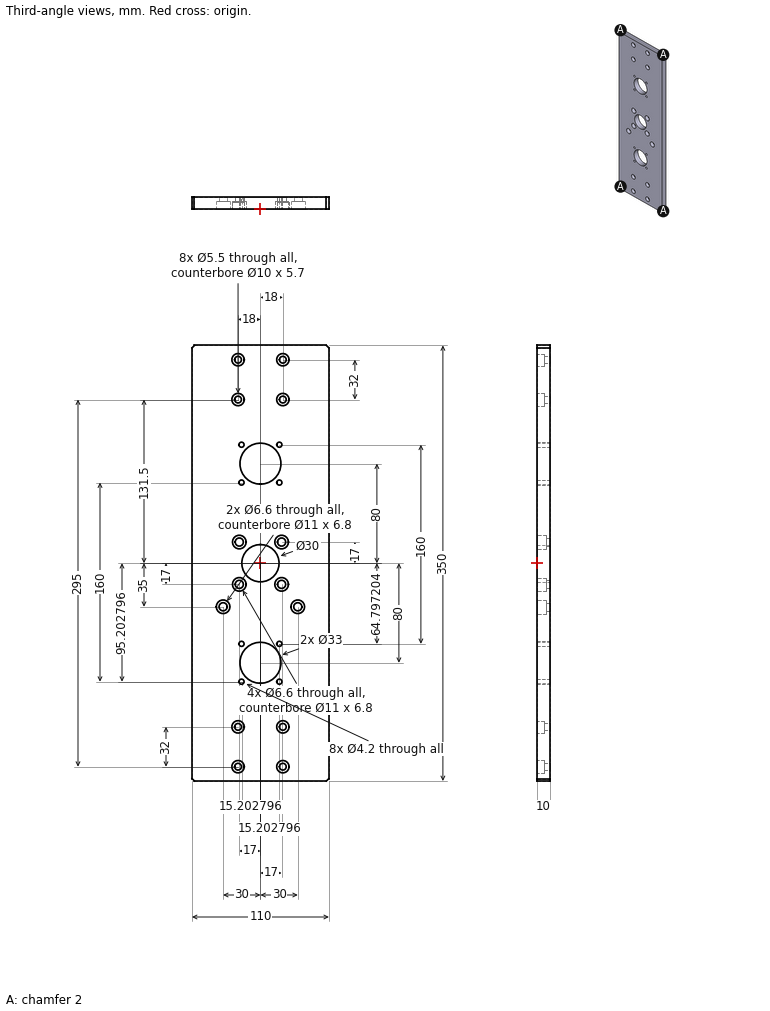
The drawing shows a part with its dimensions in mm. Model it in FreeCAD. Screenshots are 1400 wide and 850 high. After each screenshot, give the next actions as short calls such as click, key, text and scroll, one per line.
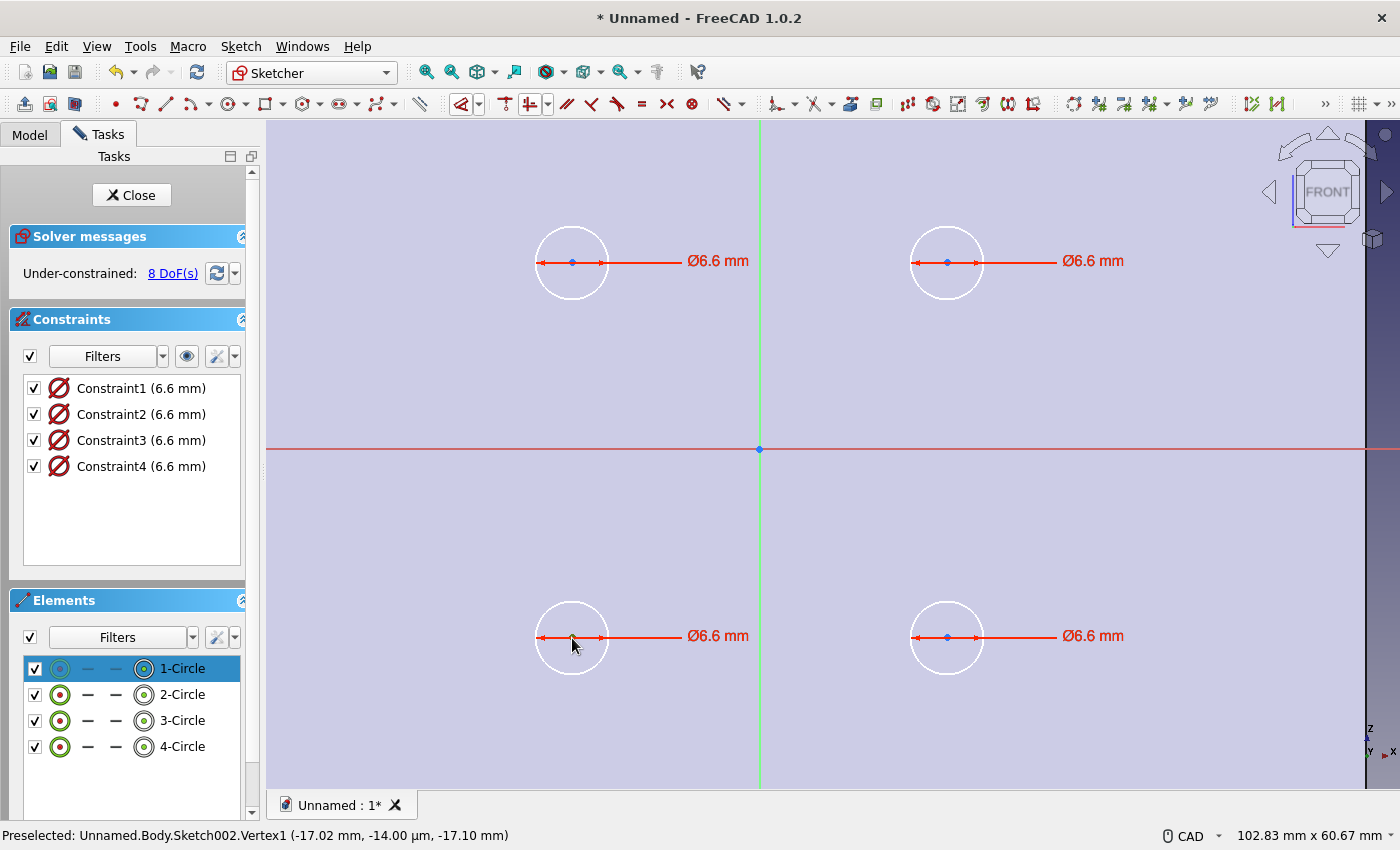
click(947, 638)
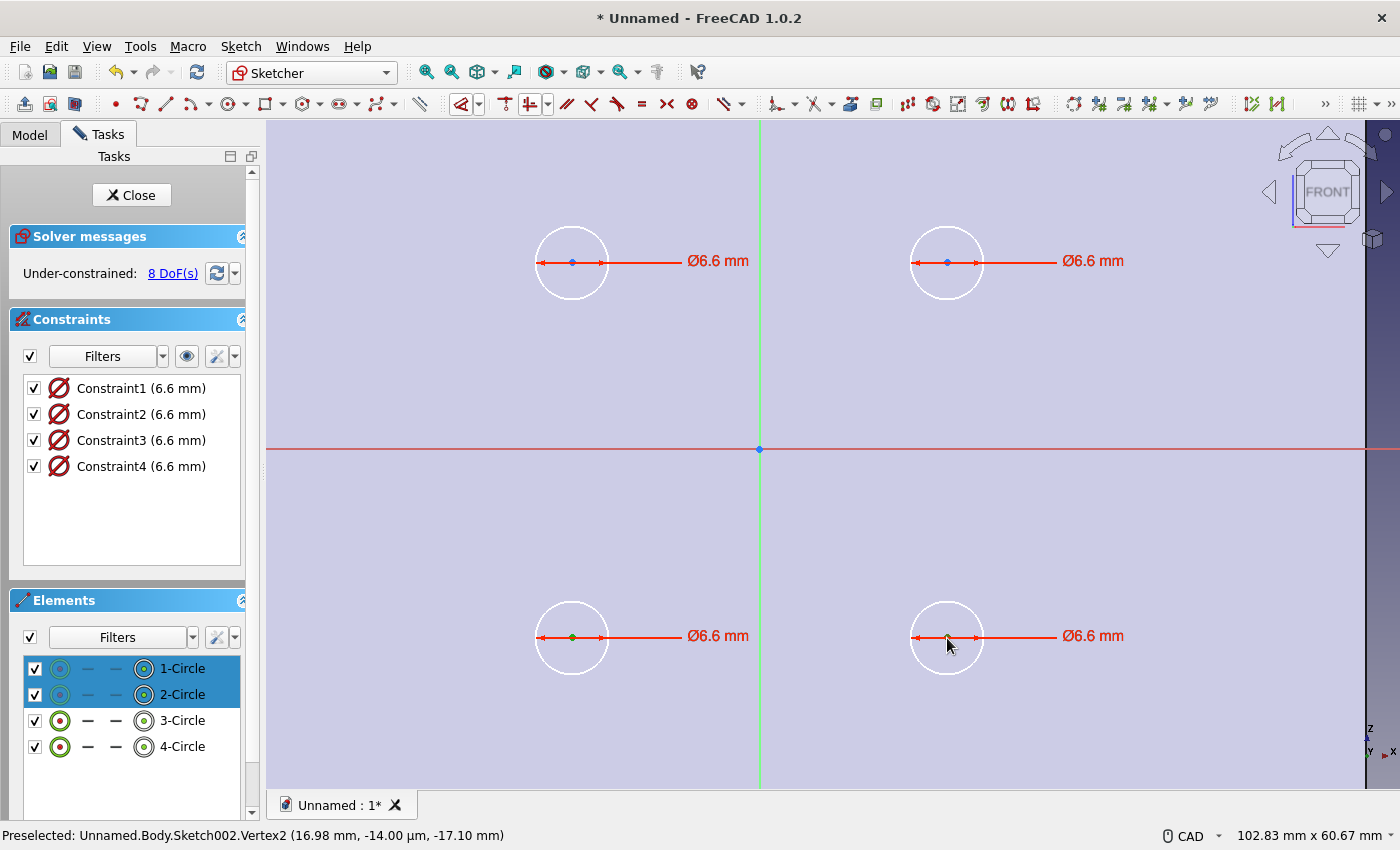
click(548, 104)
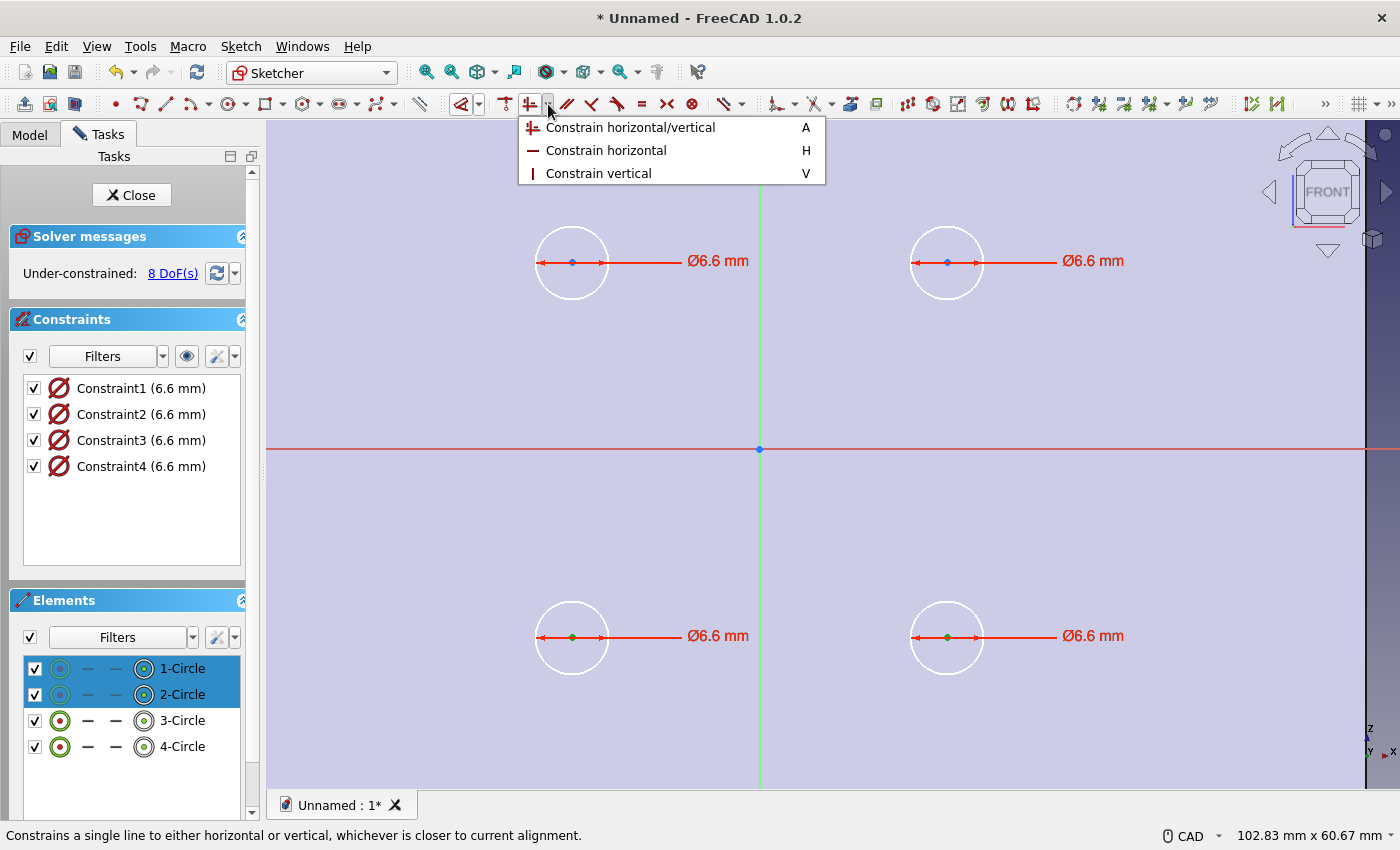
click(672, 150)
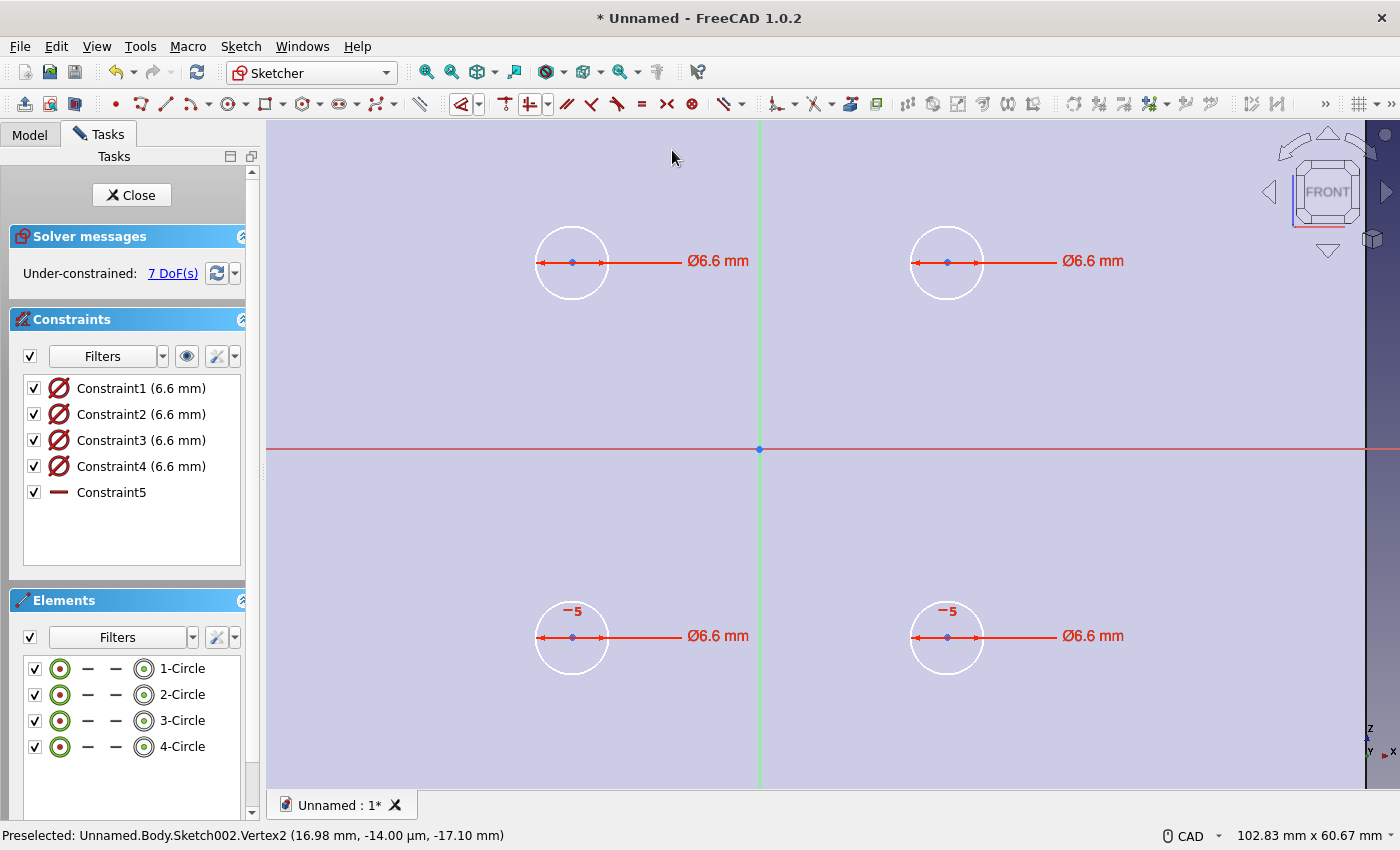
click(947, 638)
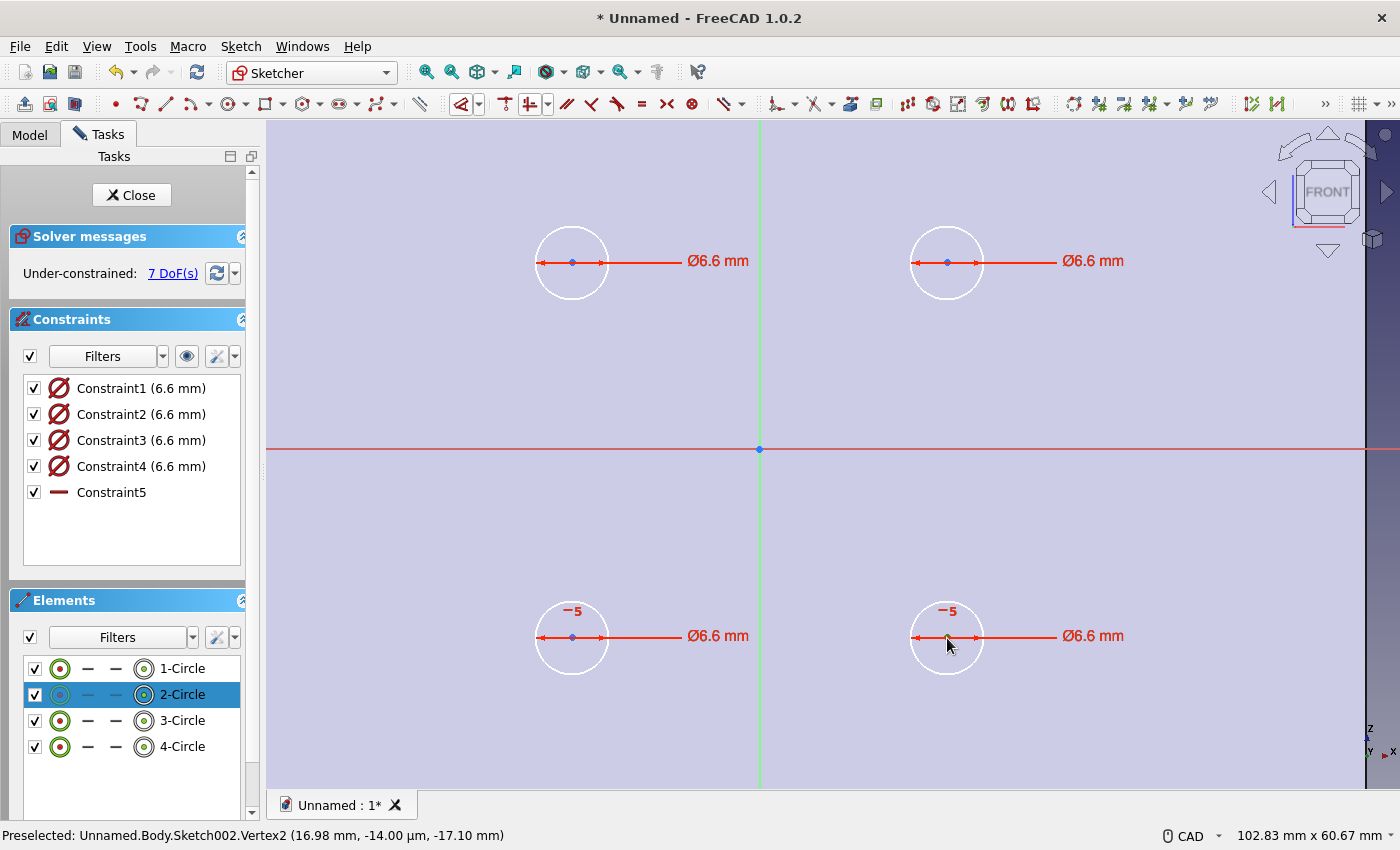
click(947, 263)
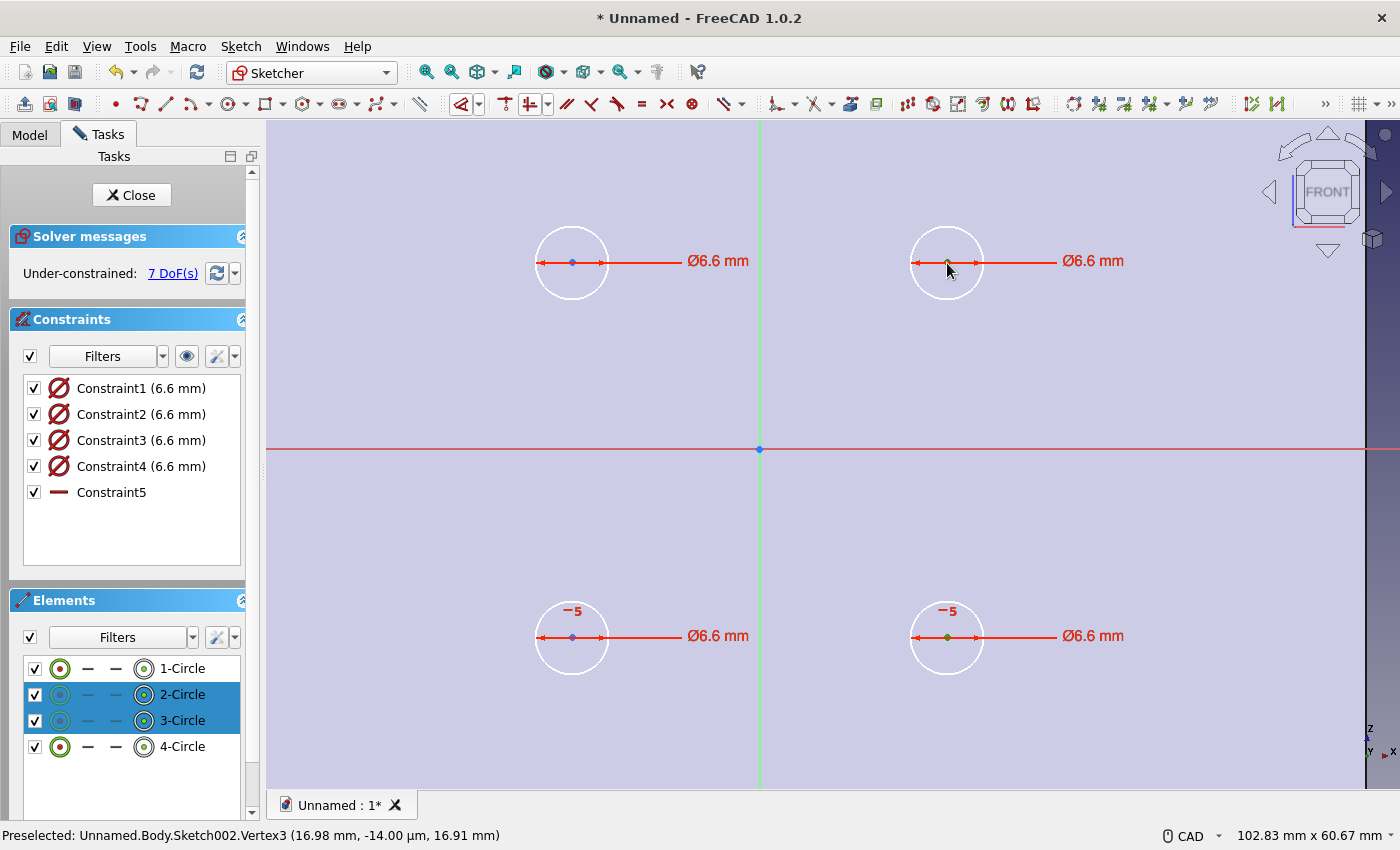
key(v)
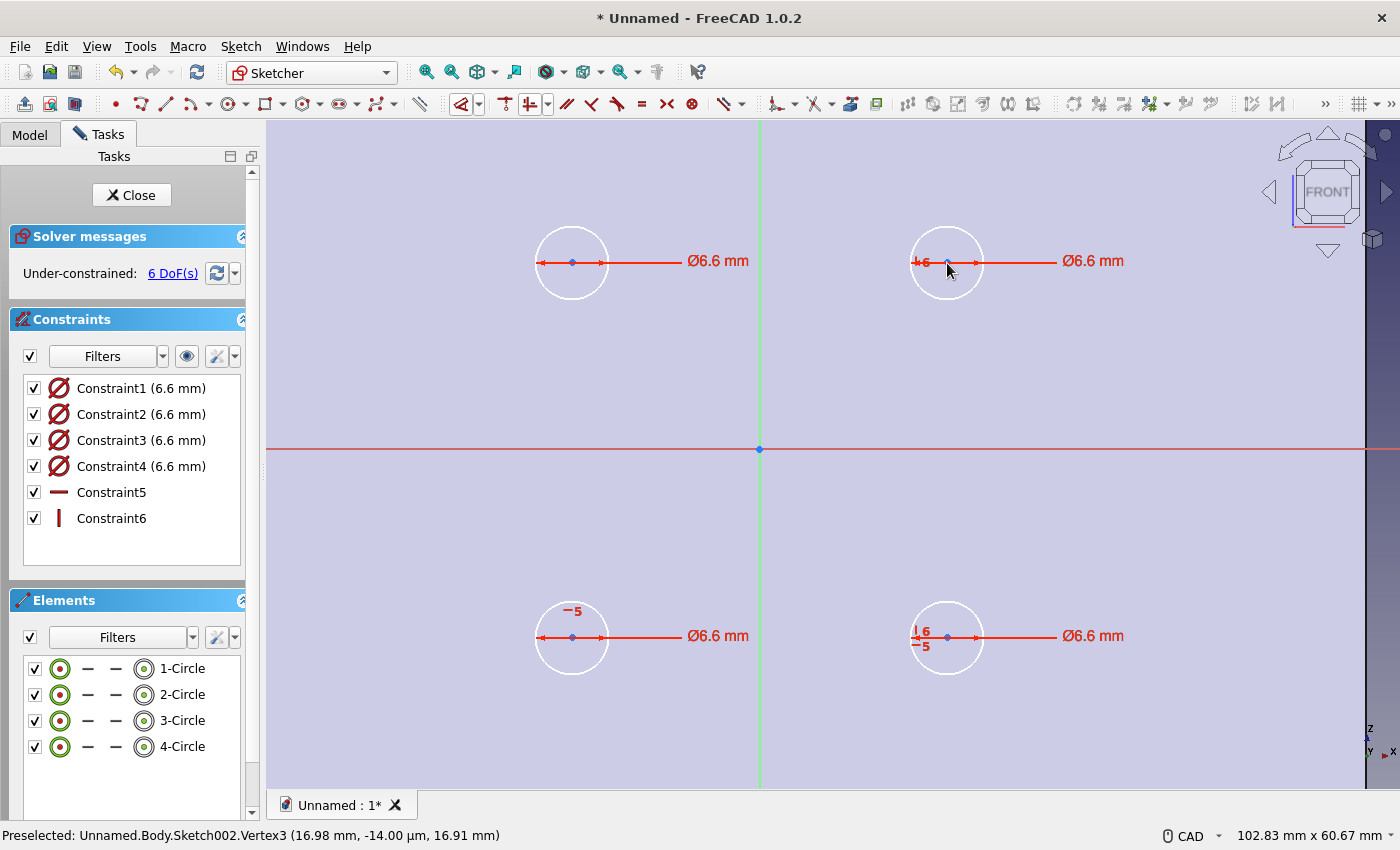
click(572, 638)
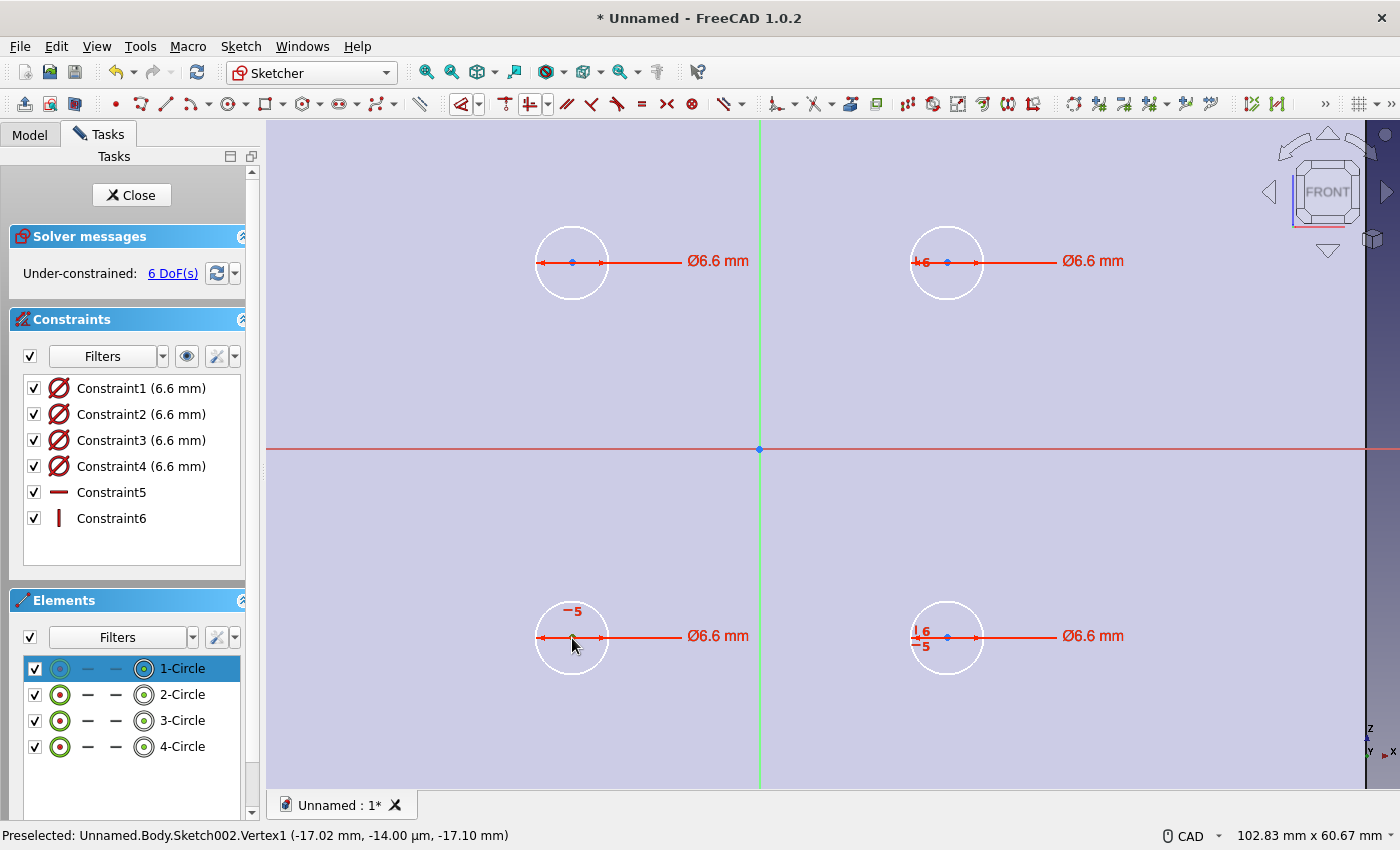
click(572, 263)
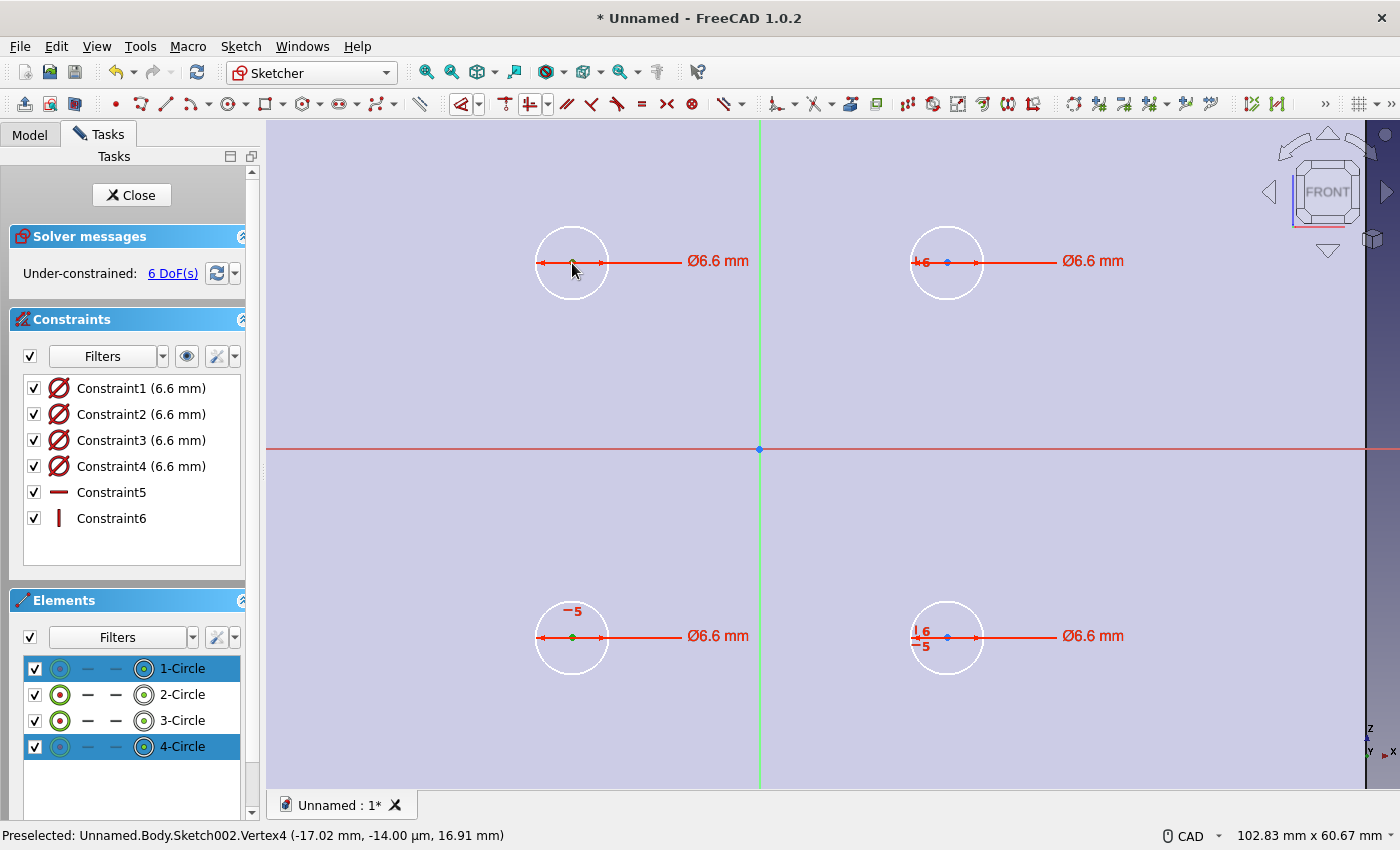
click(548, 104)